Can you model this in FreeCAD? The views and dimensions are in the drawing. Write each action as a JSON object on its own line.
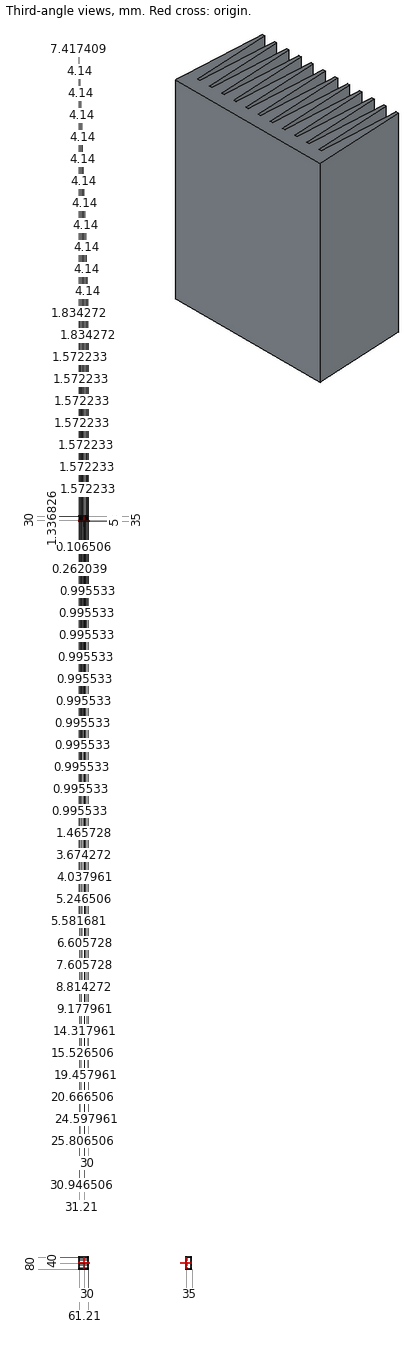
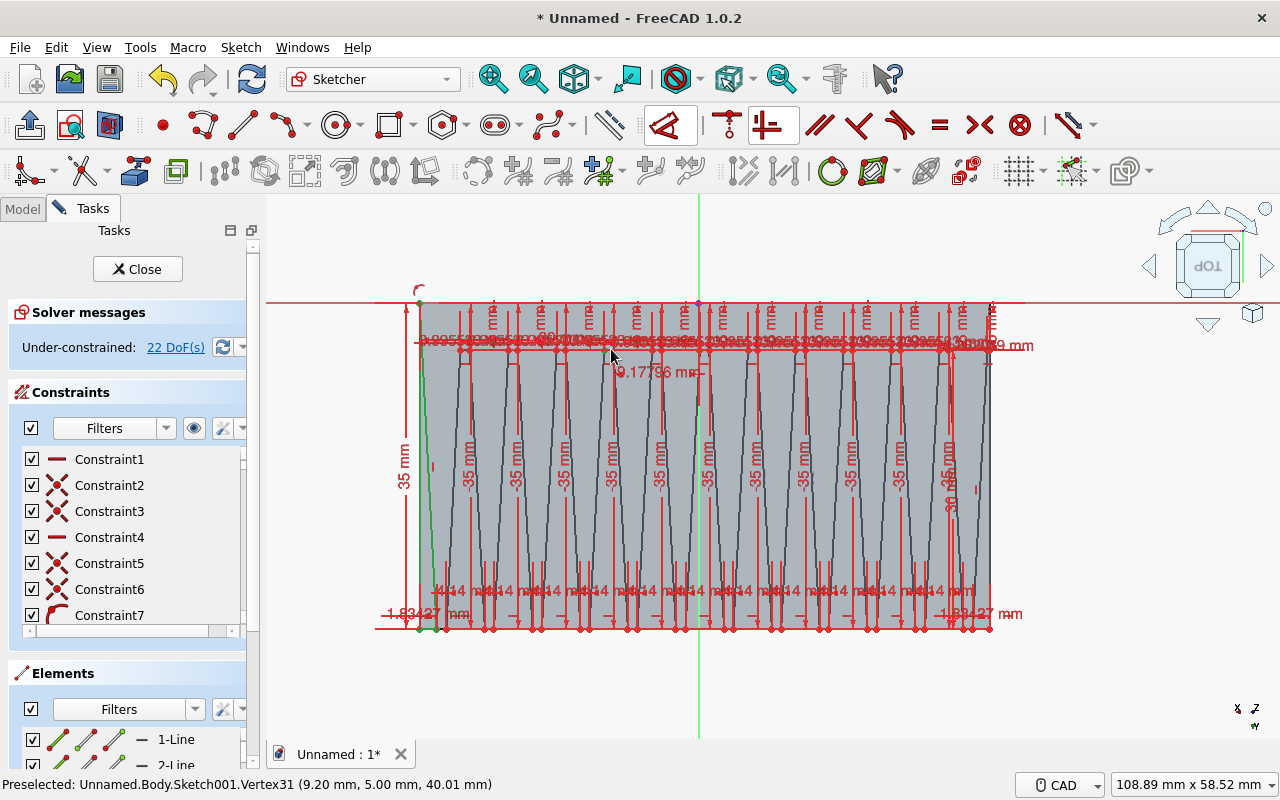
{"action": "scroll", "coordinate": [628, 629], "scroll_direction": "up", "scroll_amount": 2}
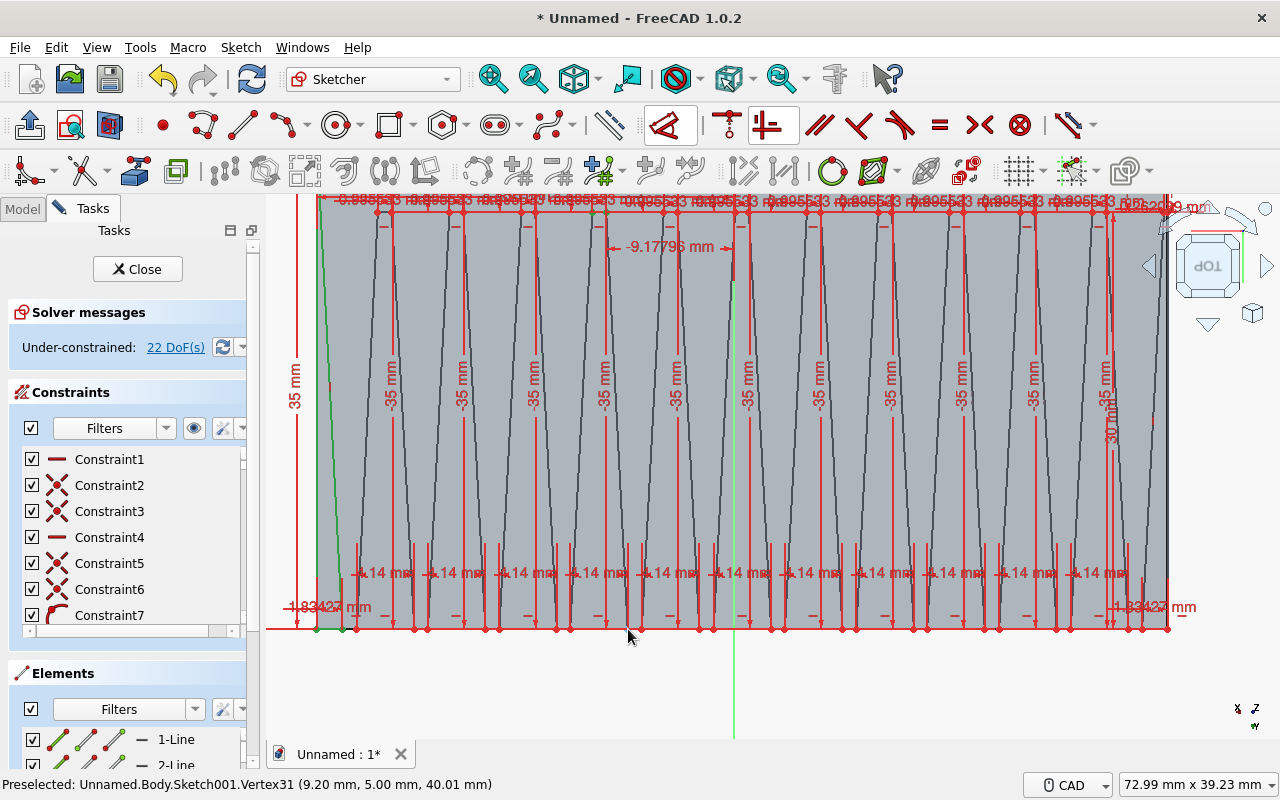
{"action": "left_click", "coordinate": [628, 629]}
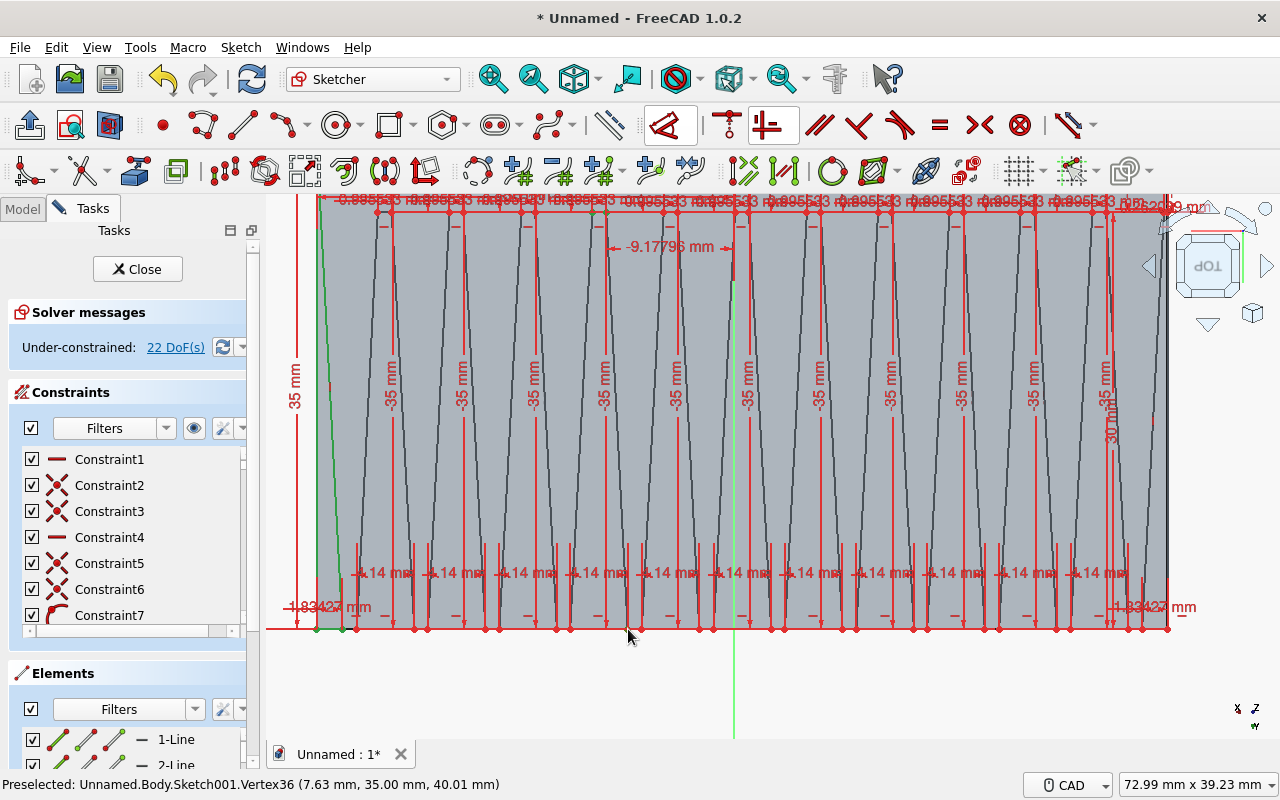
{"action": "key", "text": "l"}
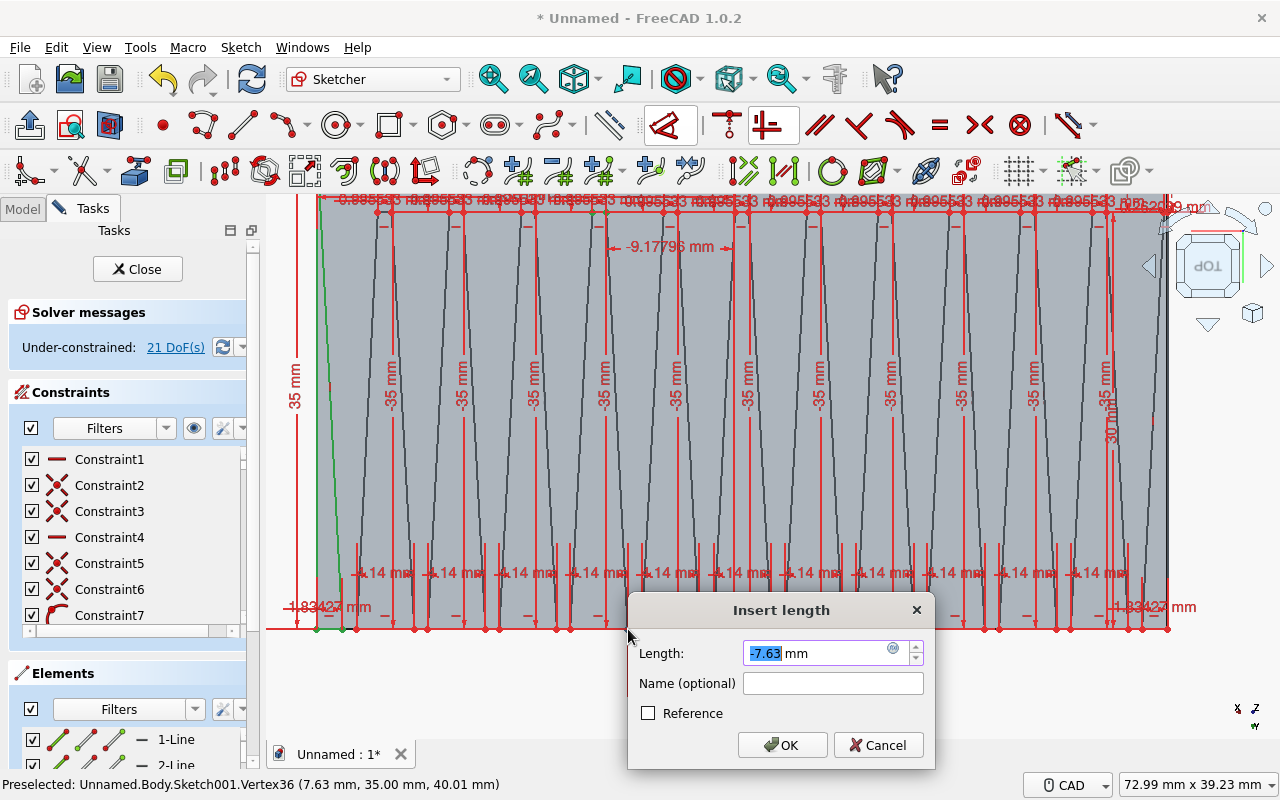
{"action": "type", "text": "-7.605728"}
{"action": "key", "text": "Return"}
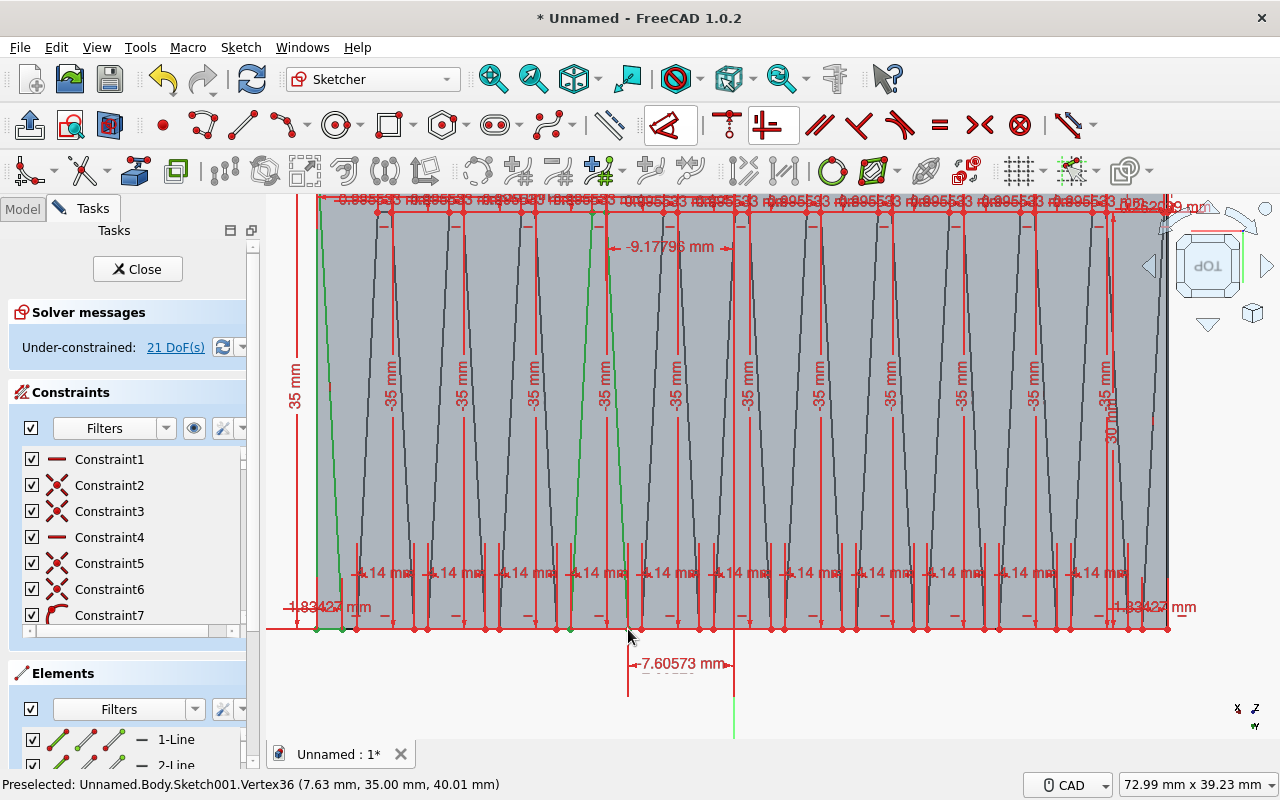
{"action": "scroll", "coordinate": [628, 630], "scroll_direction": "down", "scroll_amount": 2}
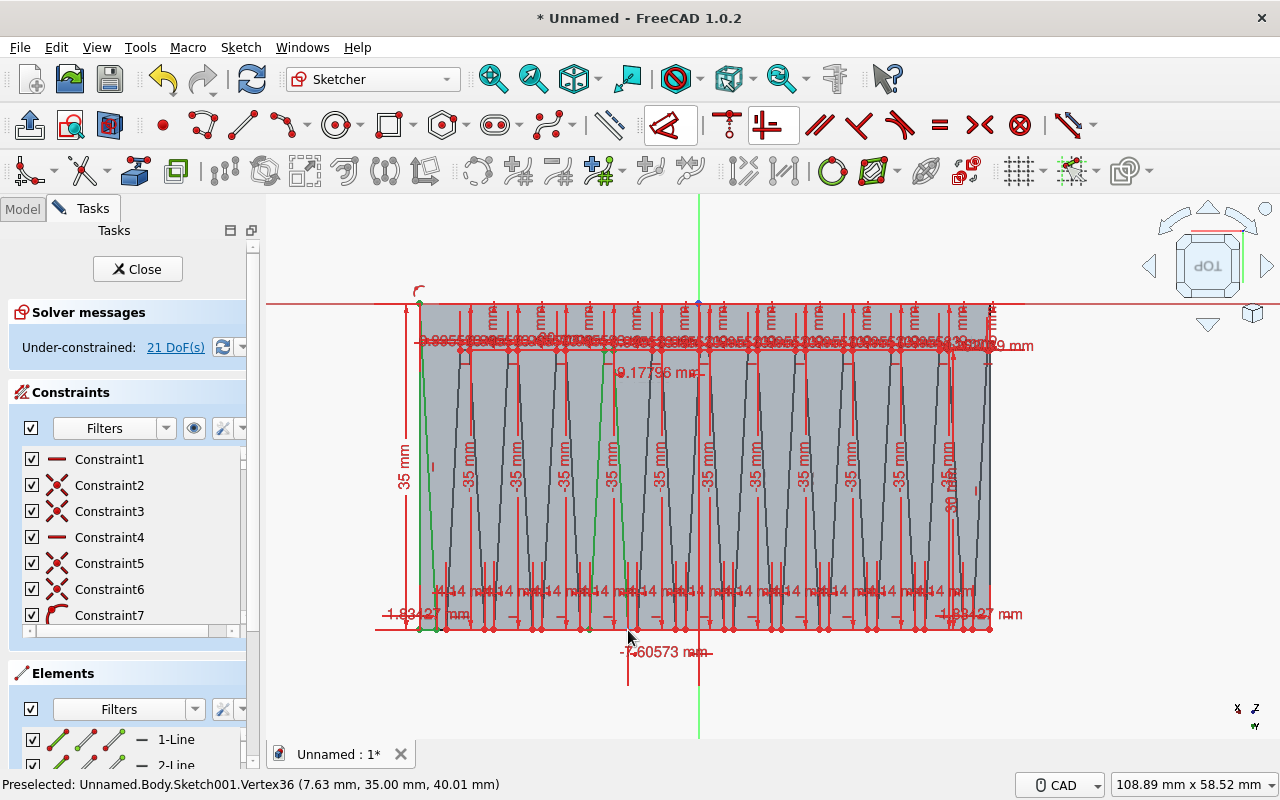
{"action": "scroll", "coordinate": [661, 350], "scroll_direction": "up", "scroll_amount": 2}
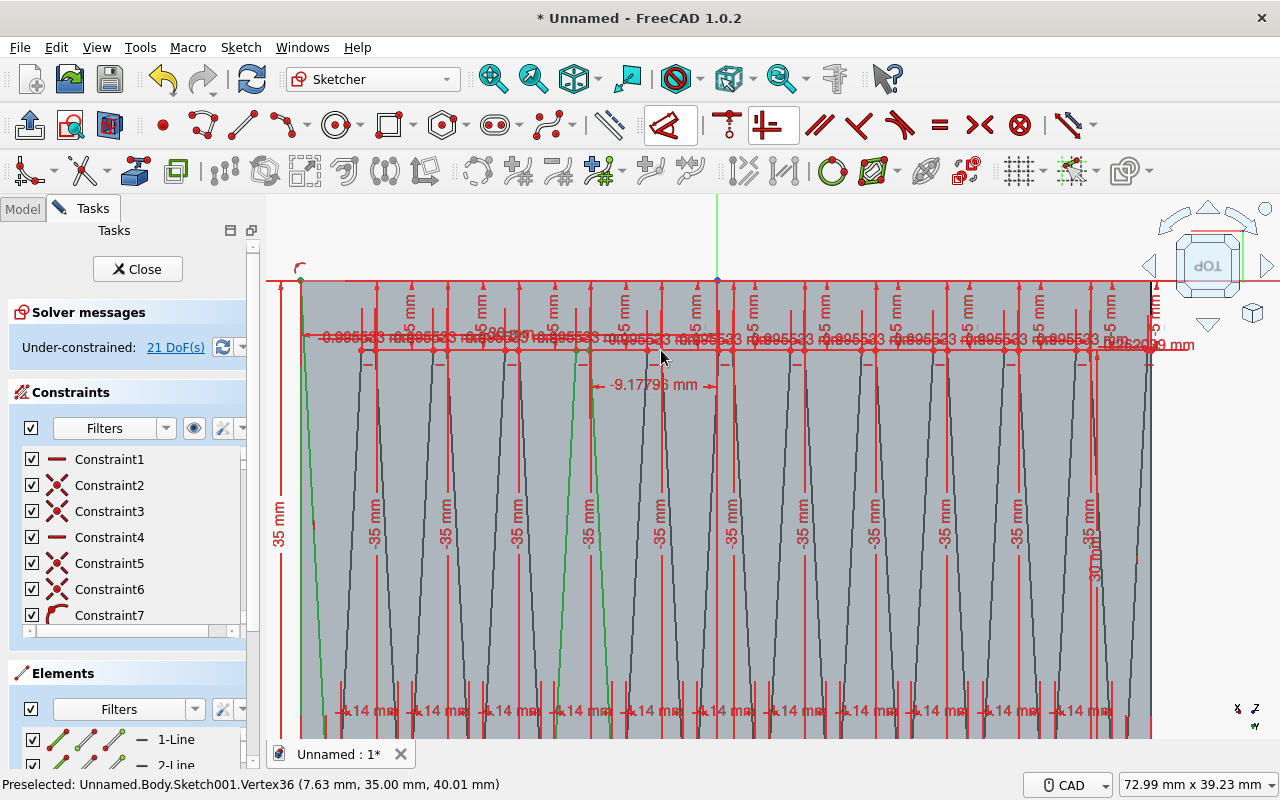
{"action": "left_click", "coordinate": [661, 350]}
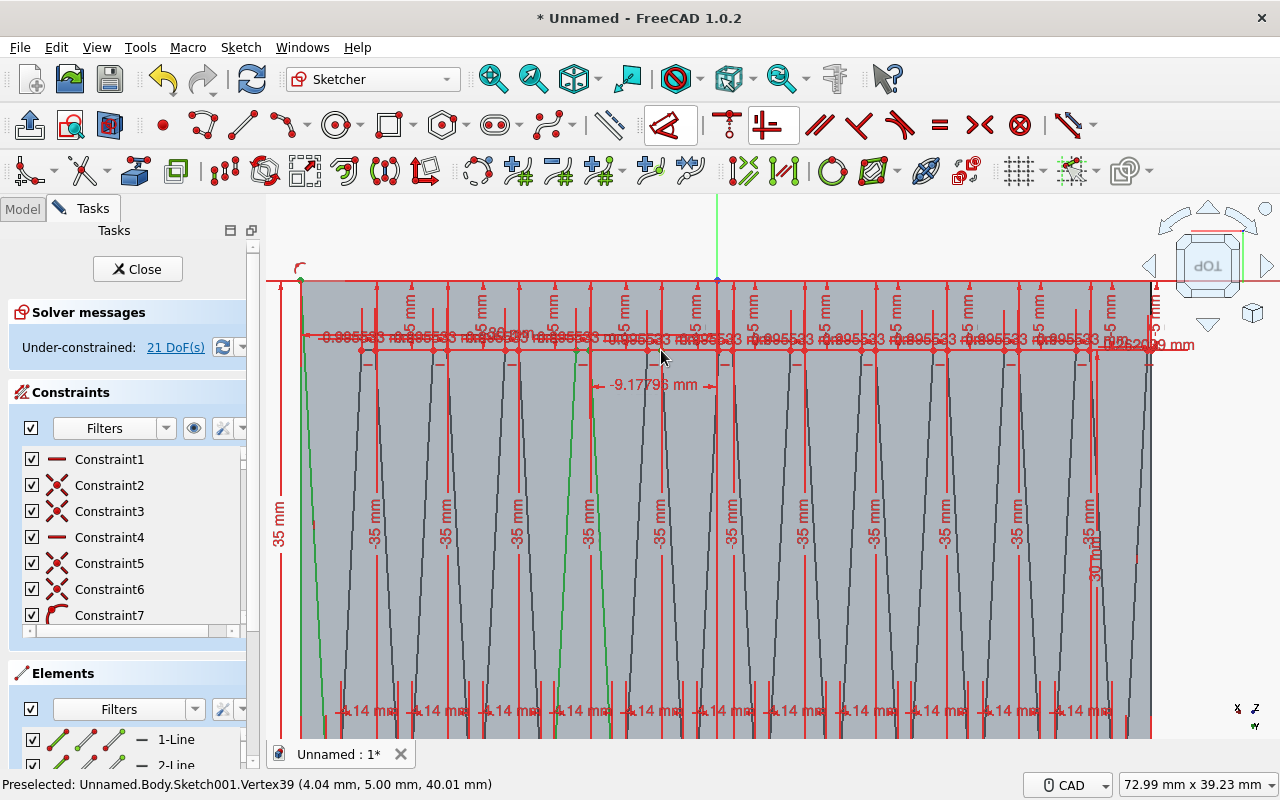
{"action": "left_click", "coordinate": [692, 126]}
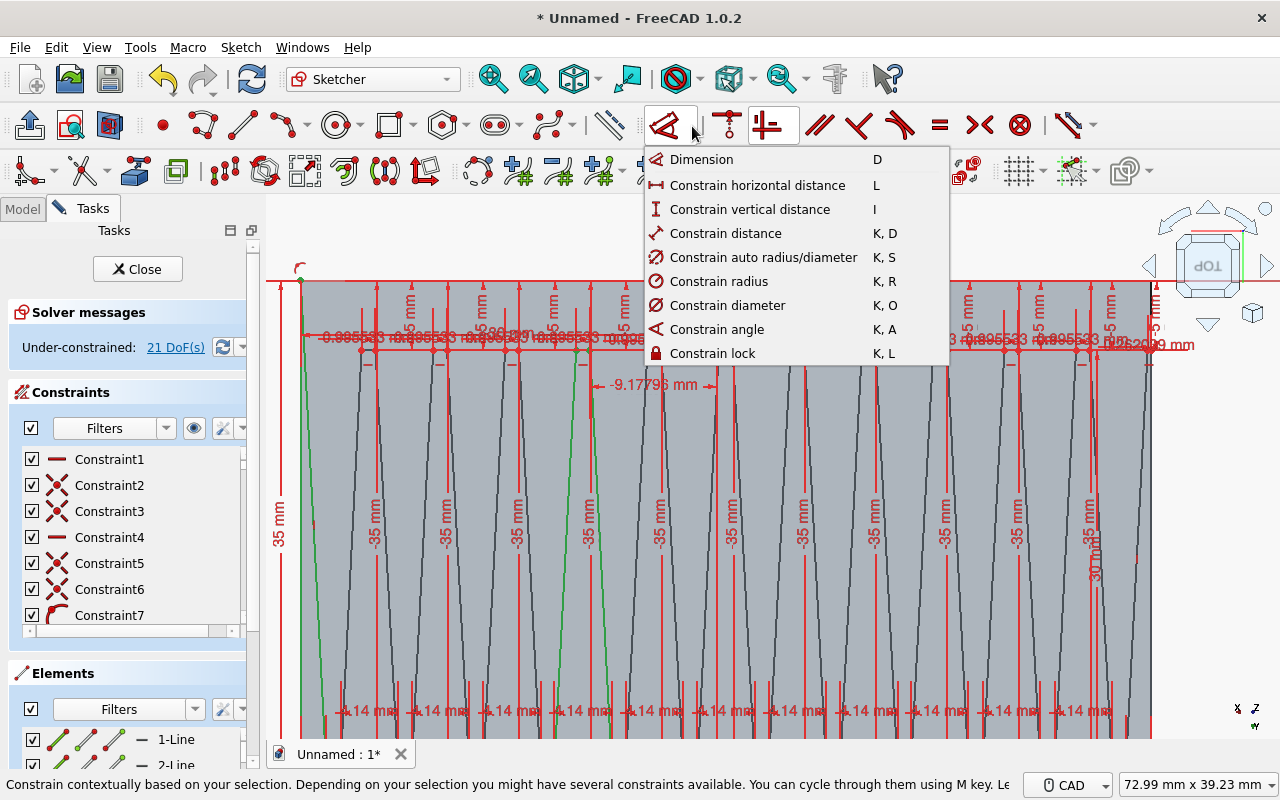
{"action": "left_click", "coordinate": [797, 185]}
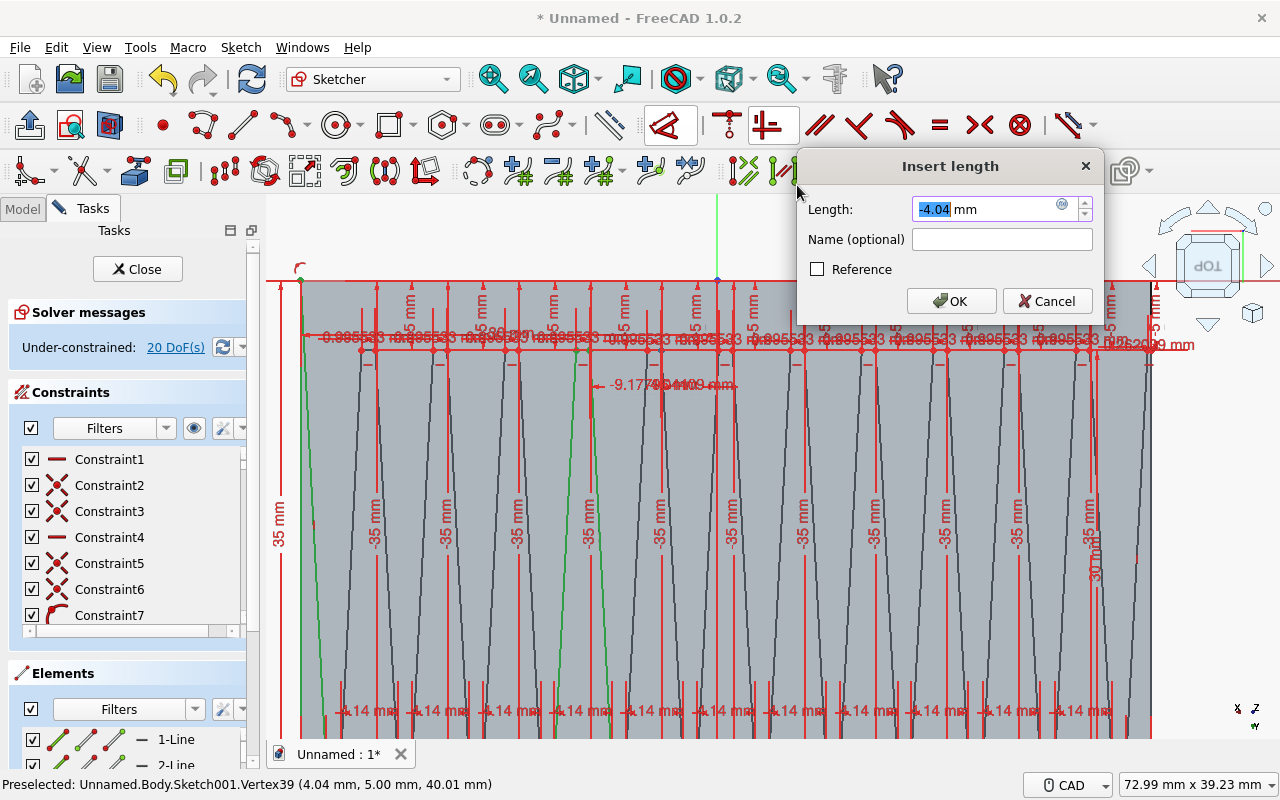
{"action": "type", "text": "-4.037961"}
{"action": "key", "text": "Return"}